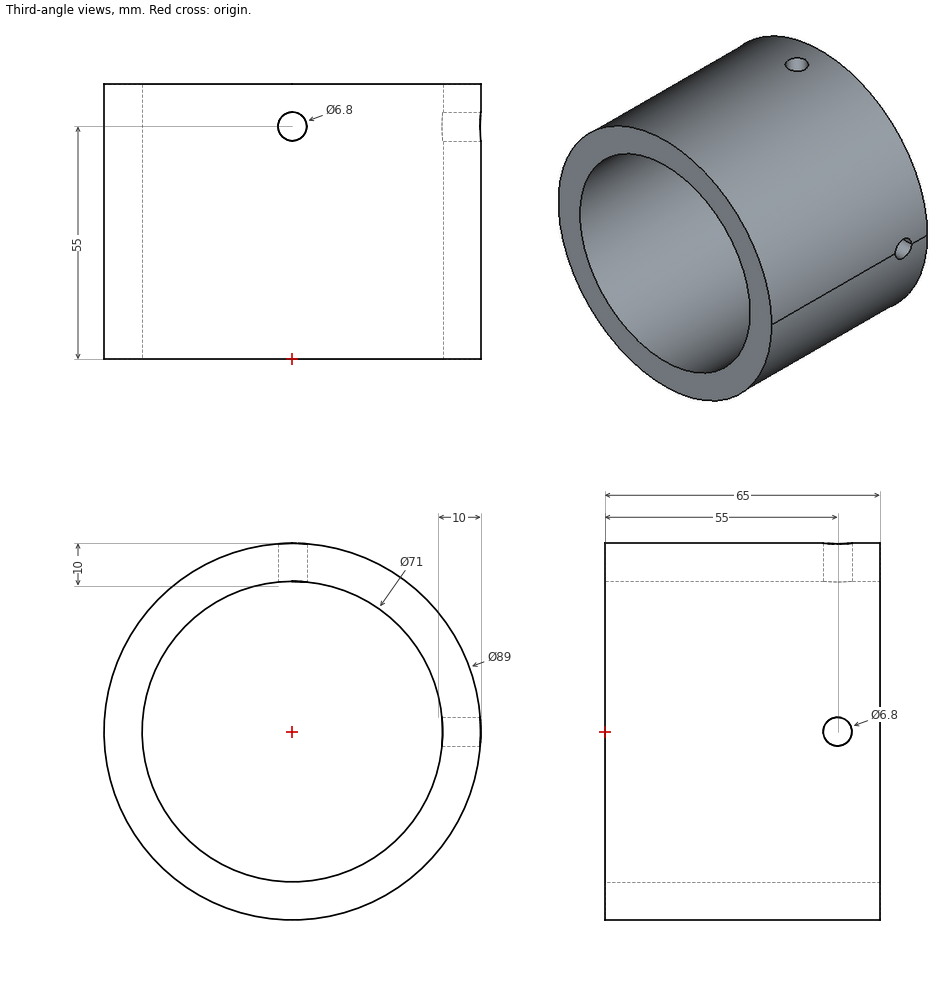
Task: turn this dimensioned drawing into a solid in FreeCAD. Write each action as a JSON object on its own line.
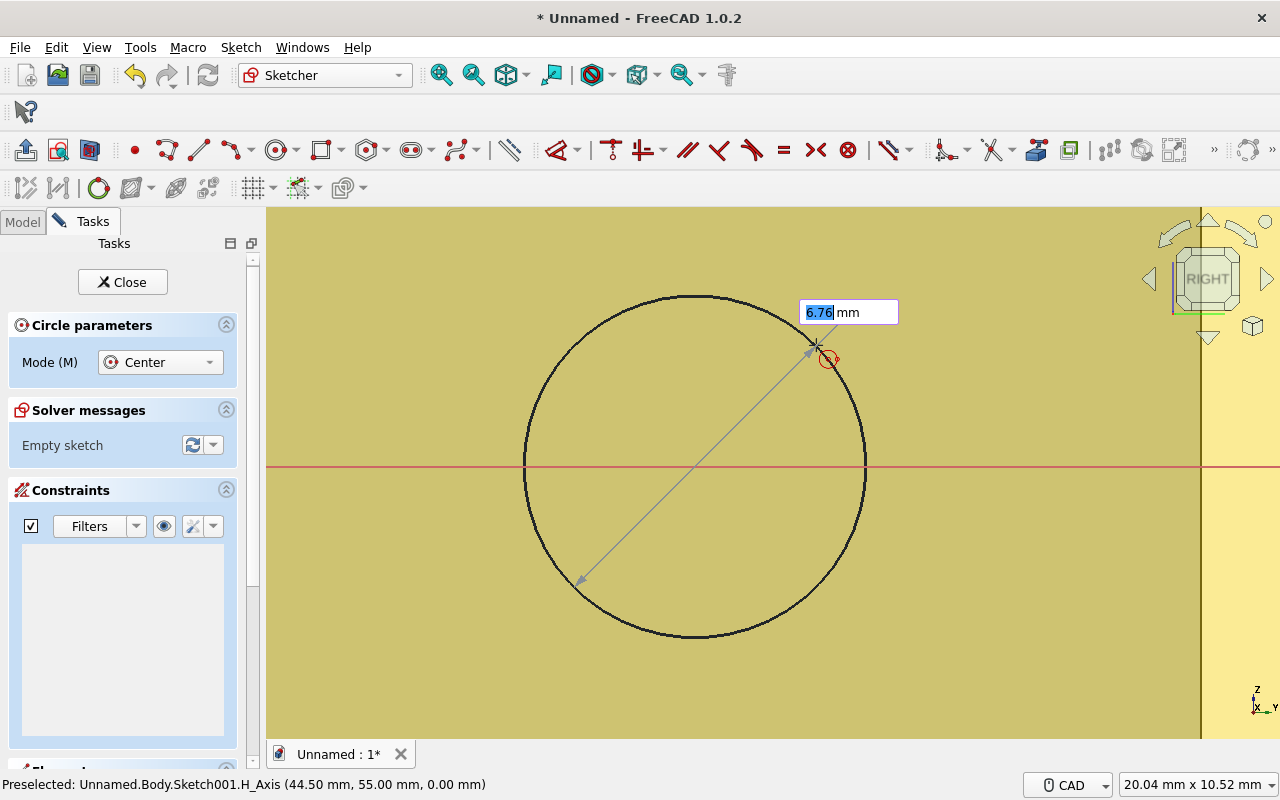
{"action": "type", "text": "6.8"}
{"action": "key", "text": "Return"}
{"action": "key", "text": "Escape"}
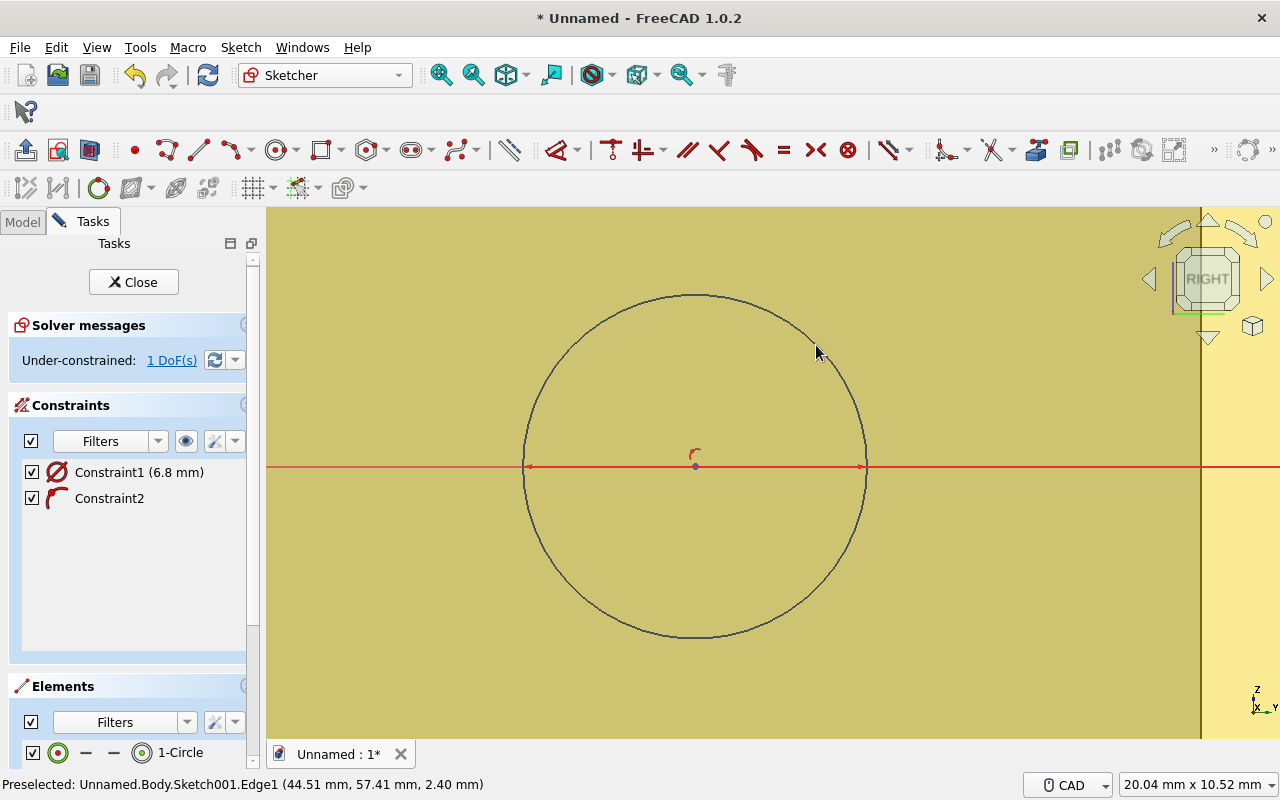
{"action": "key", "text": "d"}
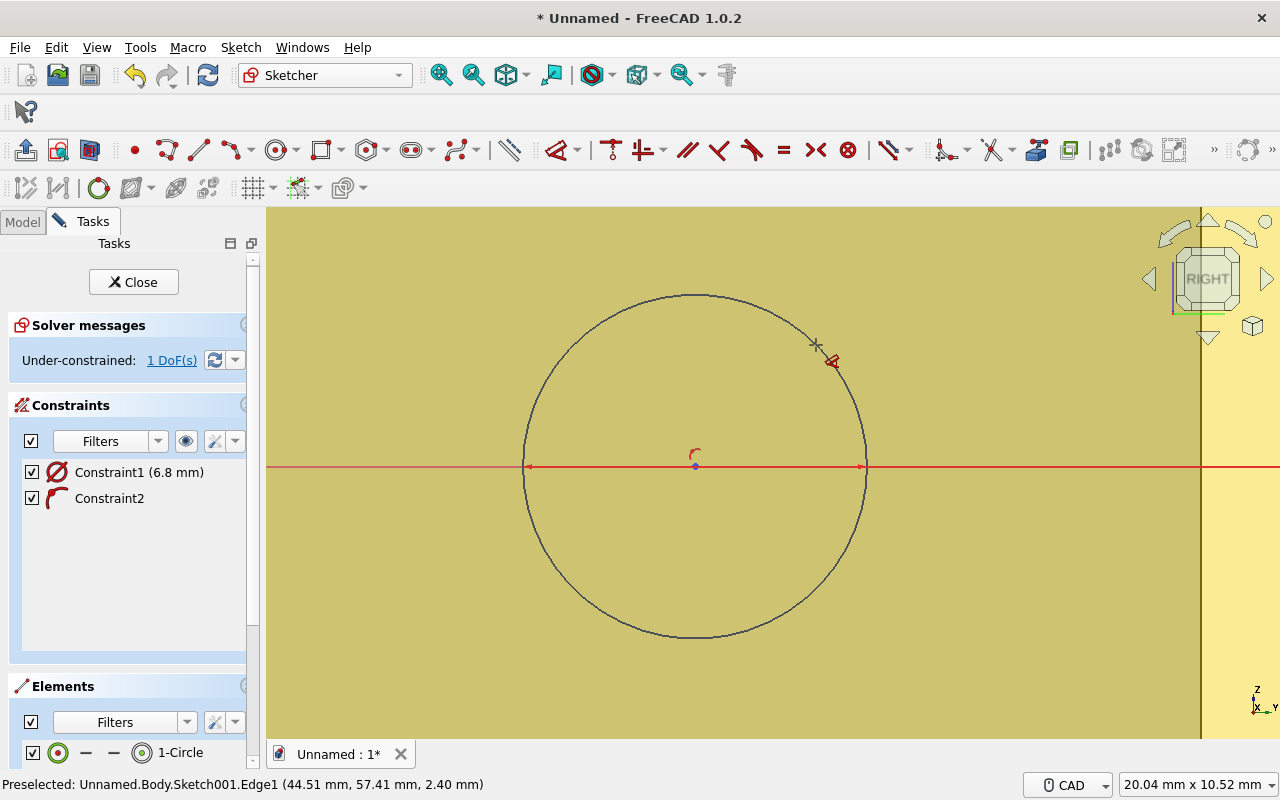
{"action": "left_click", "coordinate": [695, 467]}
{"action": "left_click", "coordinate": [495, 501]}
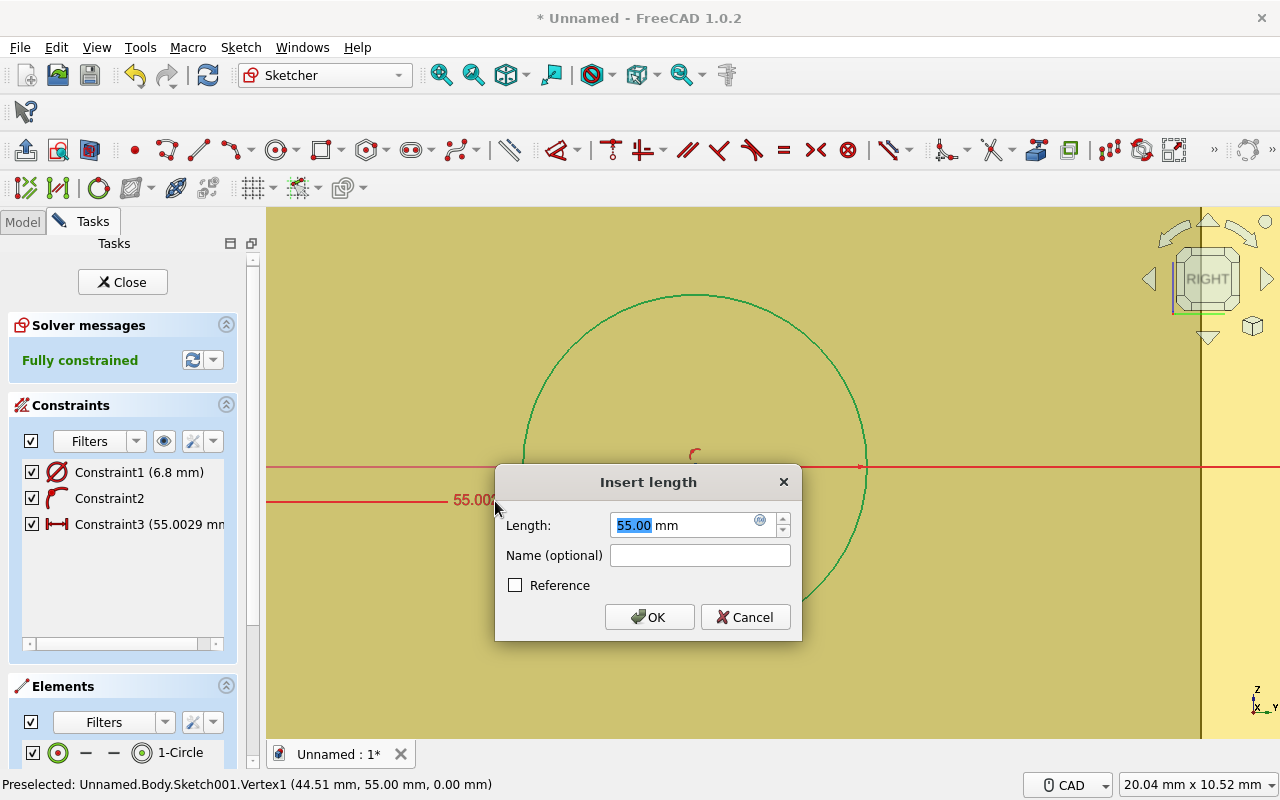
{"action": "type", "text": "55"}
{"action": "key", "text": "Return"}
{"action": "key", "text": "Escape"}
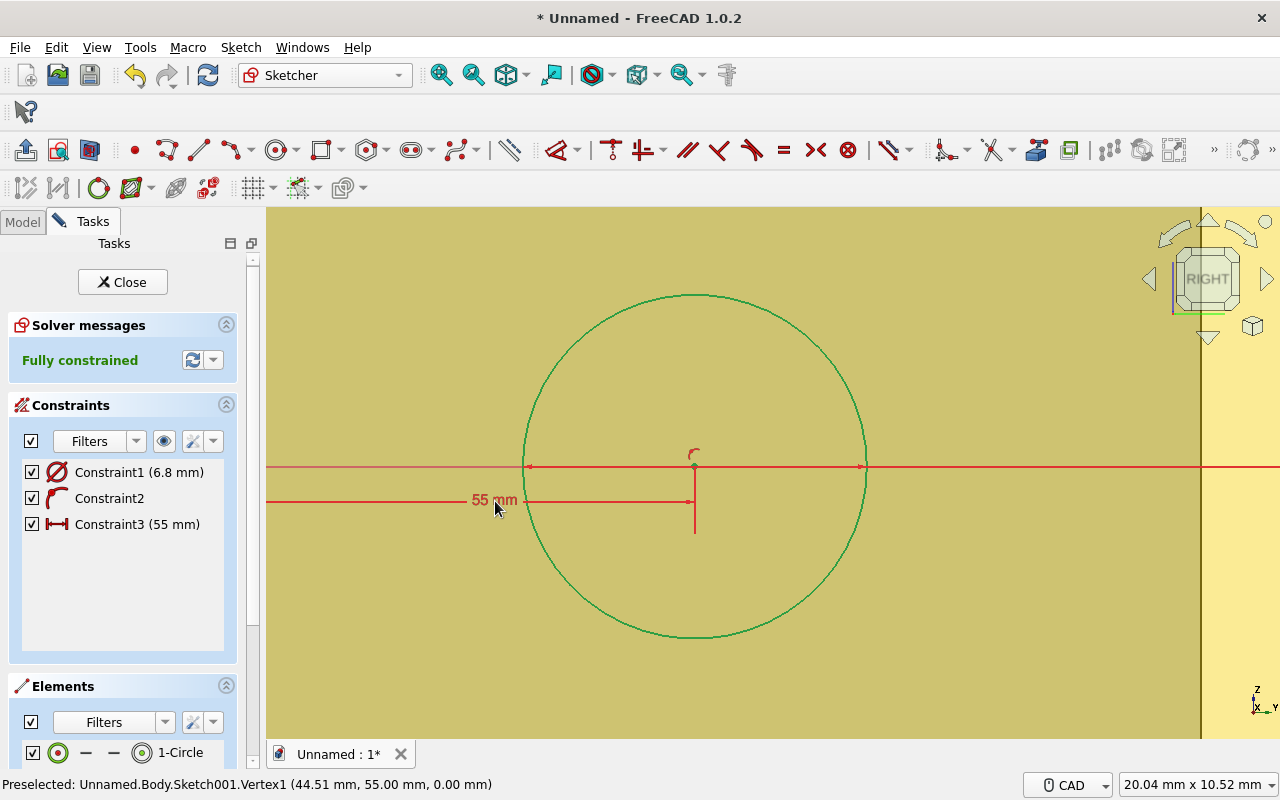
{"action": "left_click", "coordinate": [123, 282]}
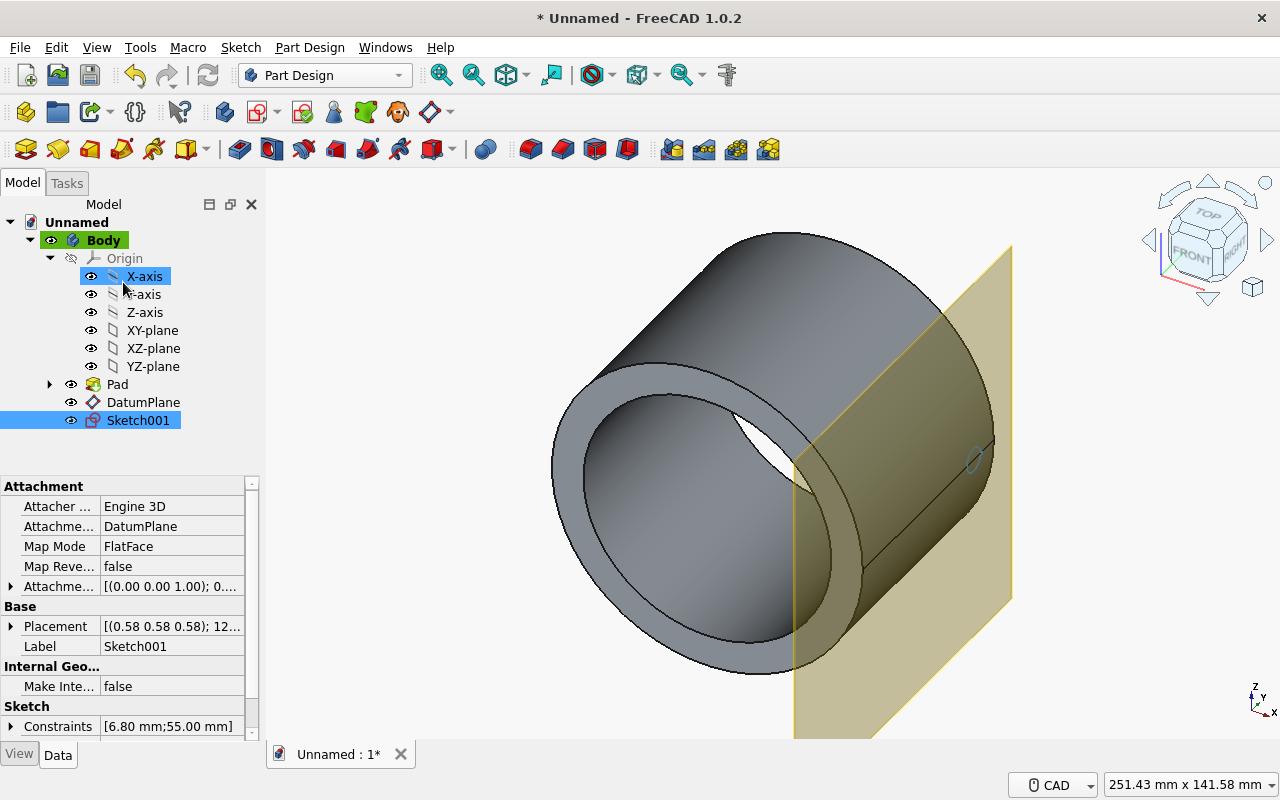
{"action": "left_click", "coordinate": [240, 150]}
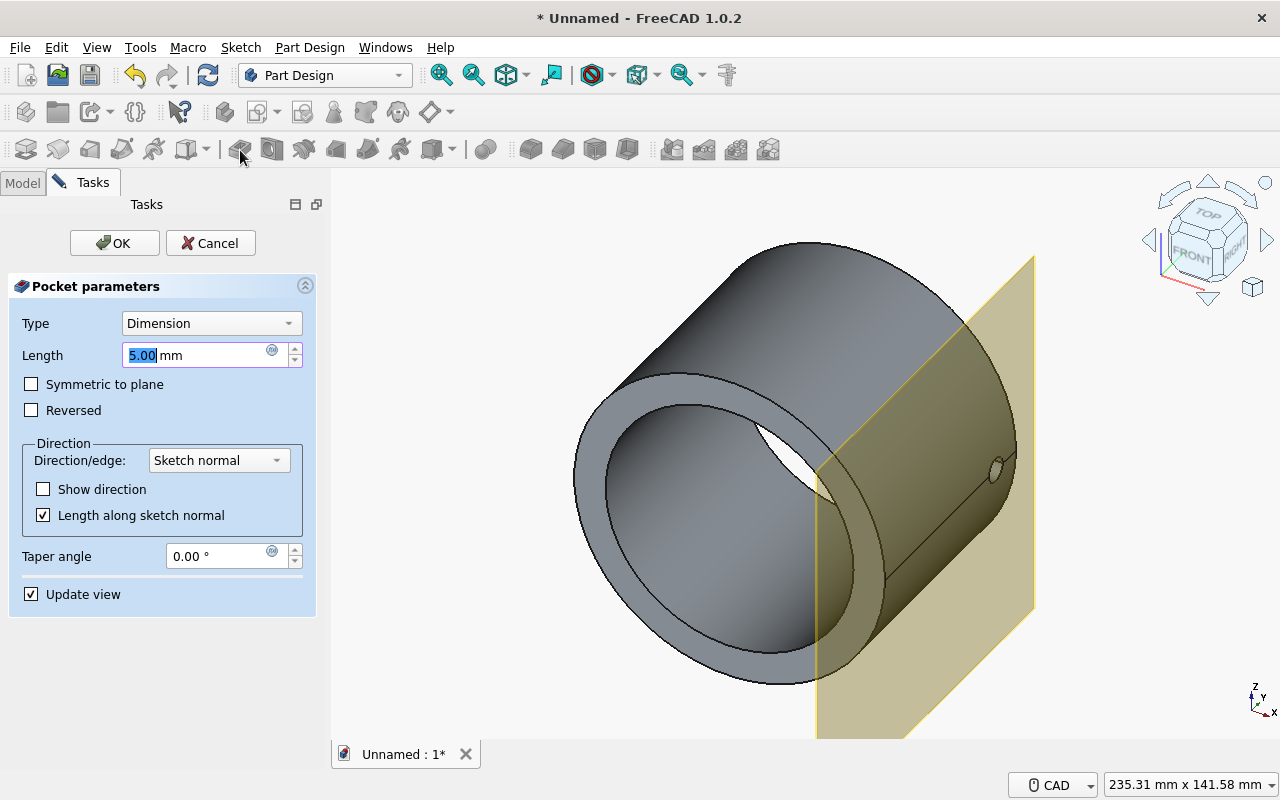
{"action": "type", "text": "10"}
{"action": "key", "text": "Tab"}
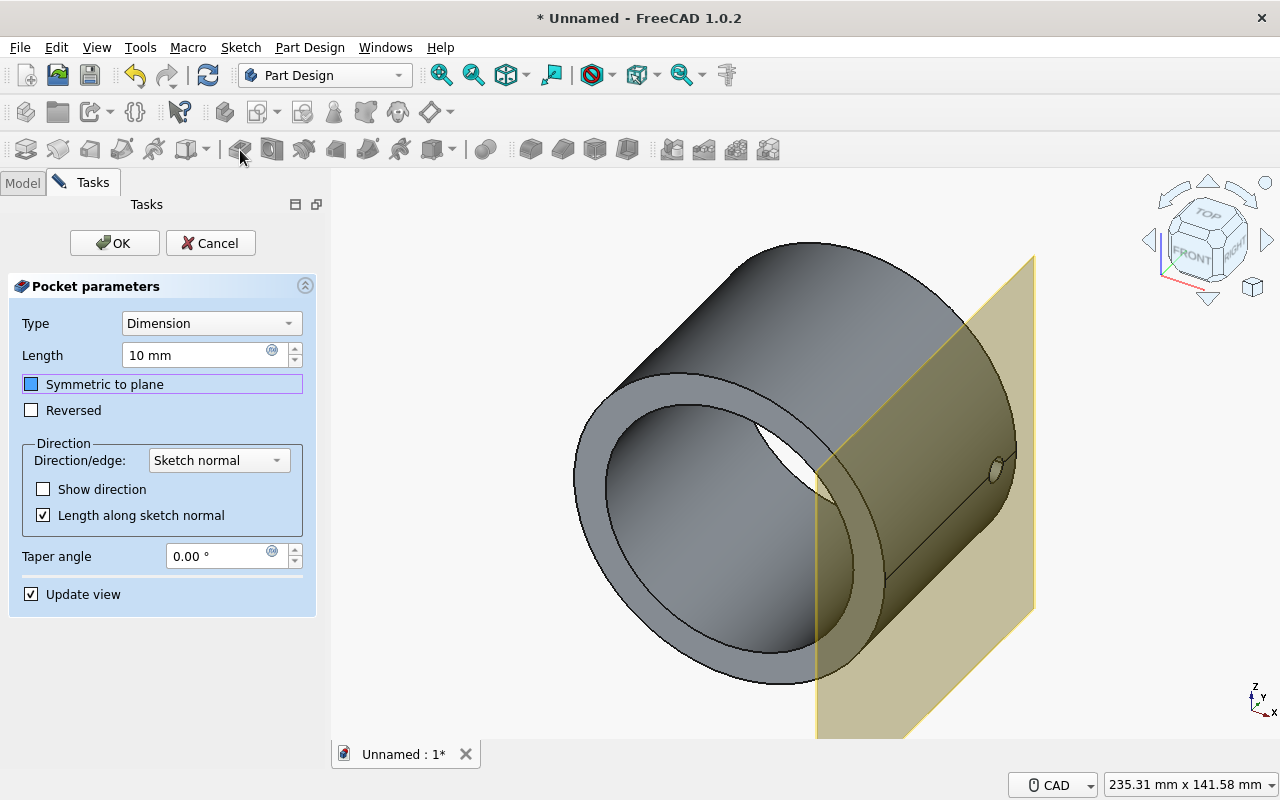
{"action": "left_click", "coordinate": [115, 243]}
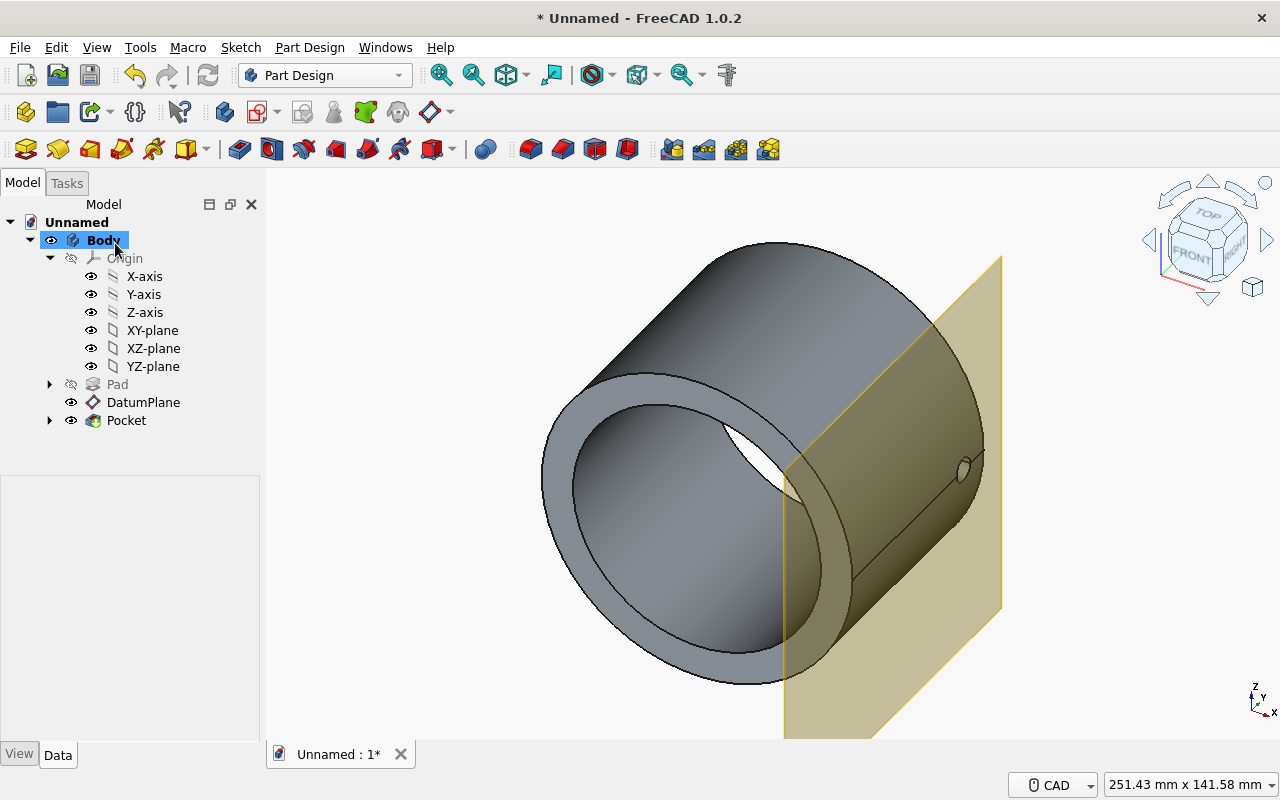
{"action": "left_click", "coordinate": [116, 402]}
{"action": "key", "text": "space"}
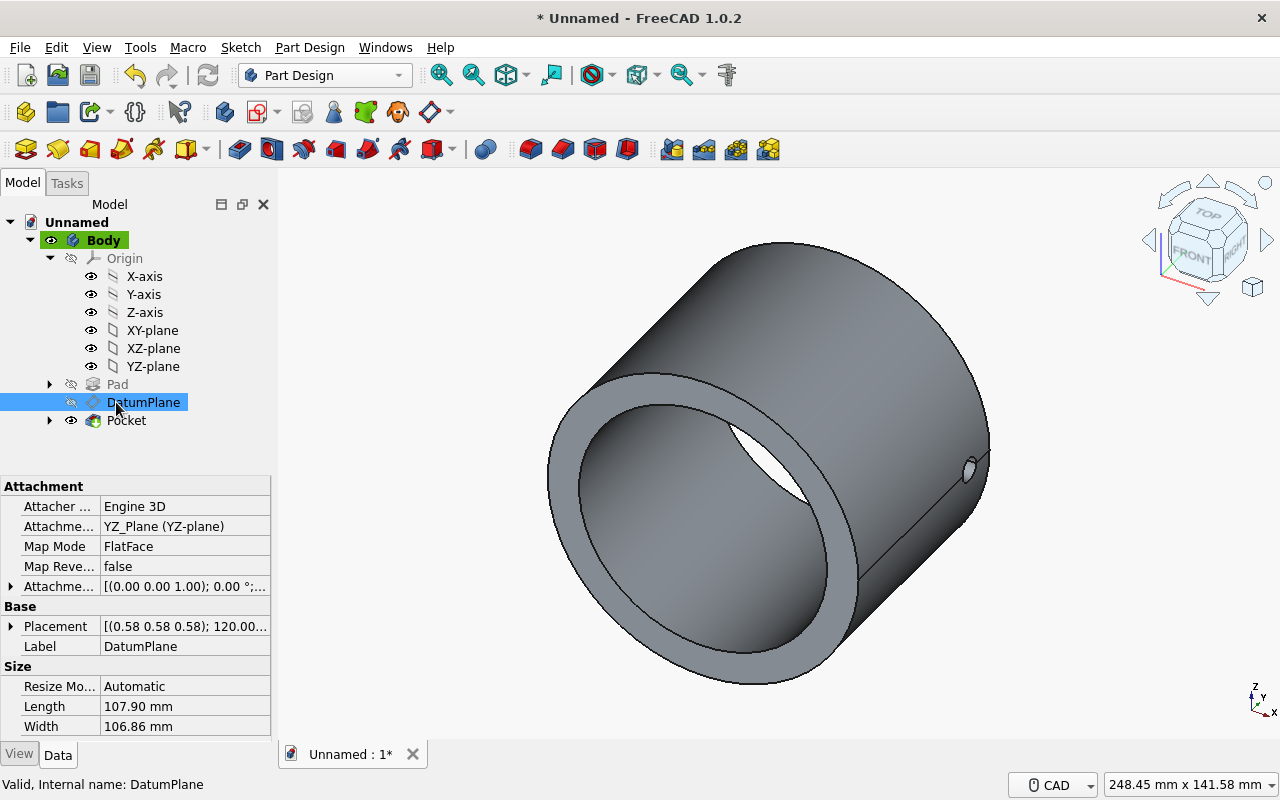
{"action": "left_click", "coordinate": [136, 330]}